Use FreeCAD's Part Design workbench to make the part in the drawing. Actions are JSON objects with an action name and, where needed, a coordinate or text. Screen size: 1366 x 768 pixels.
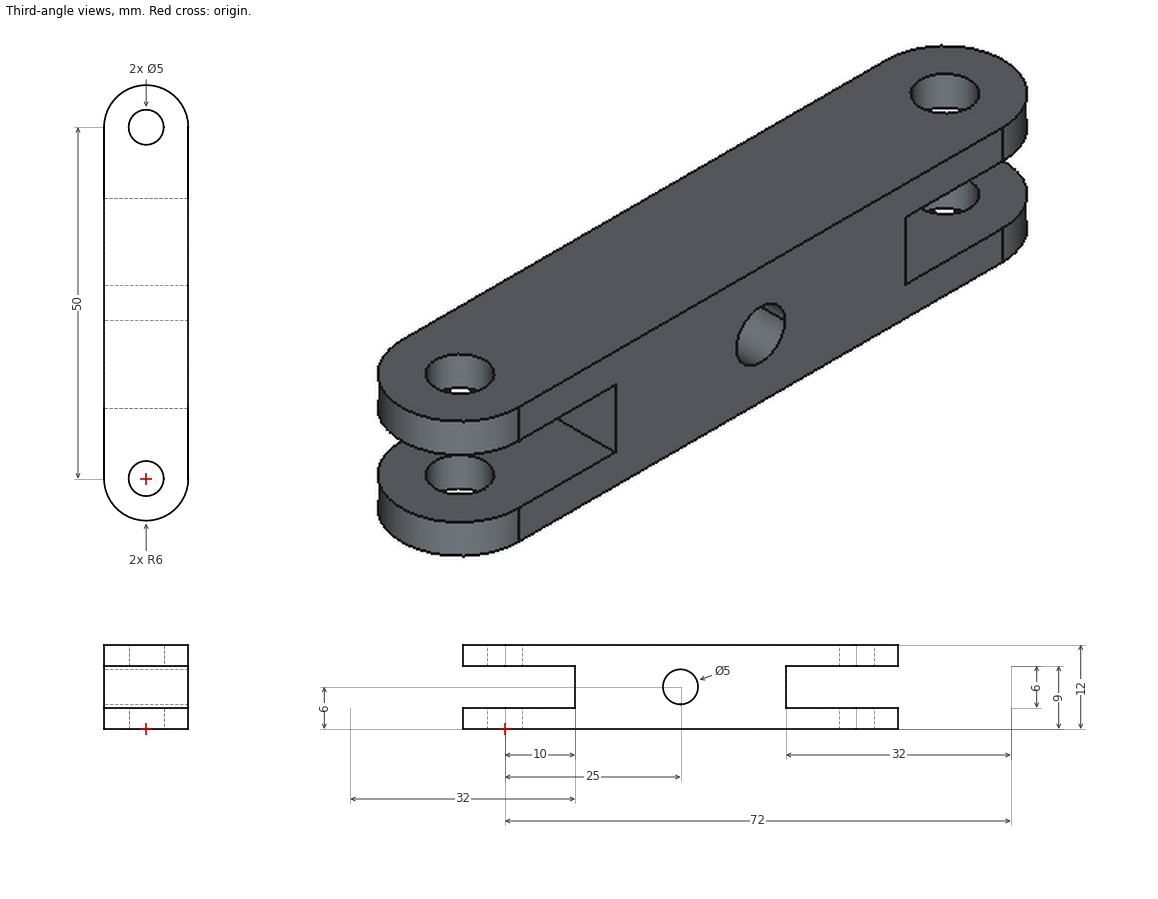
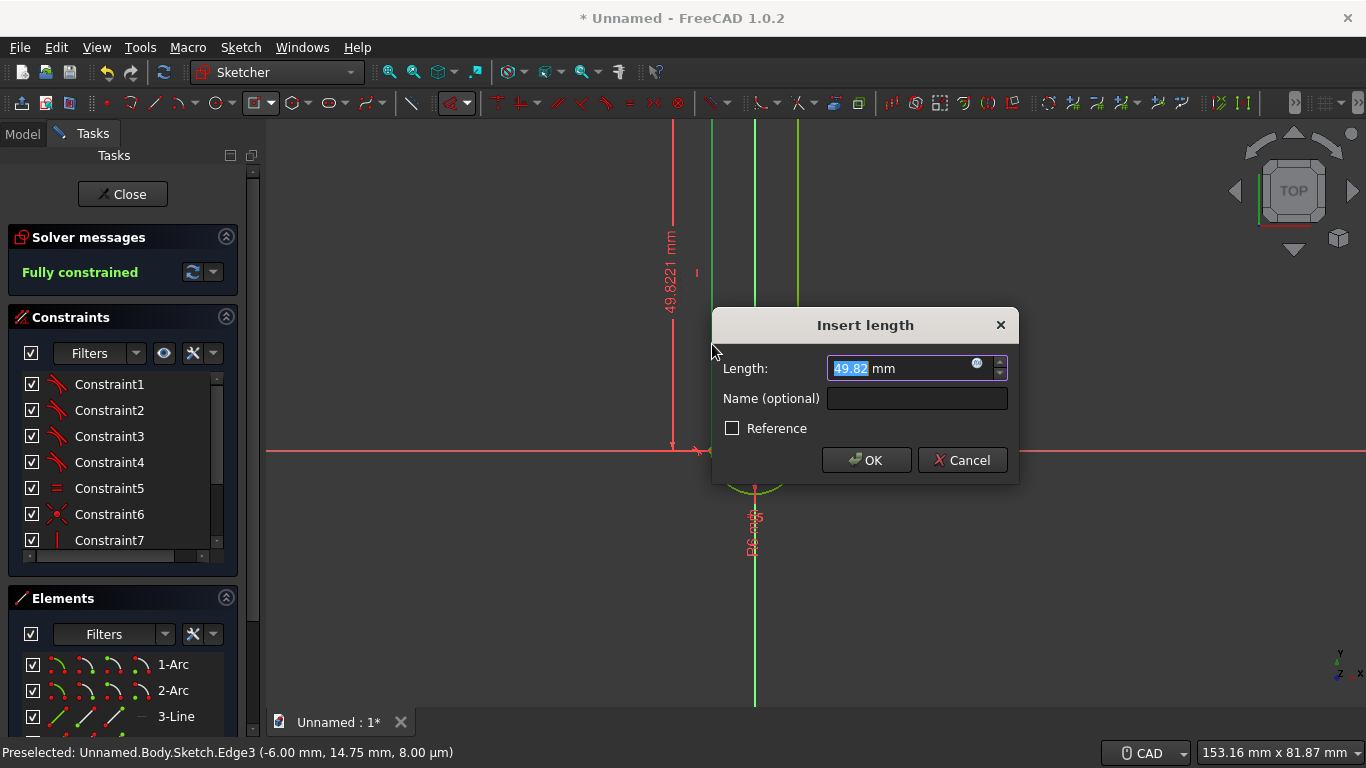
{"action": "type", "text": "50"}
{"action": "key", "text": "Return"}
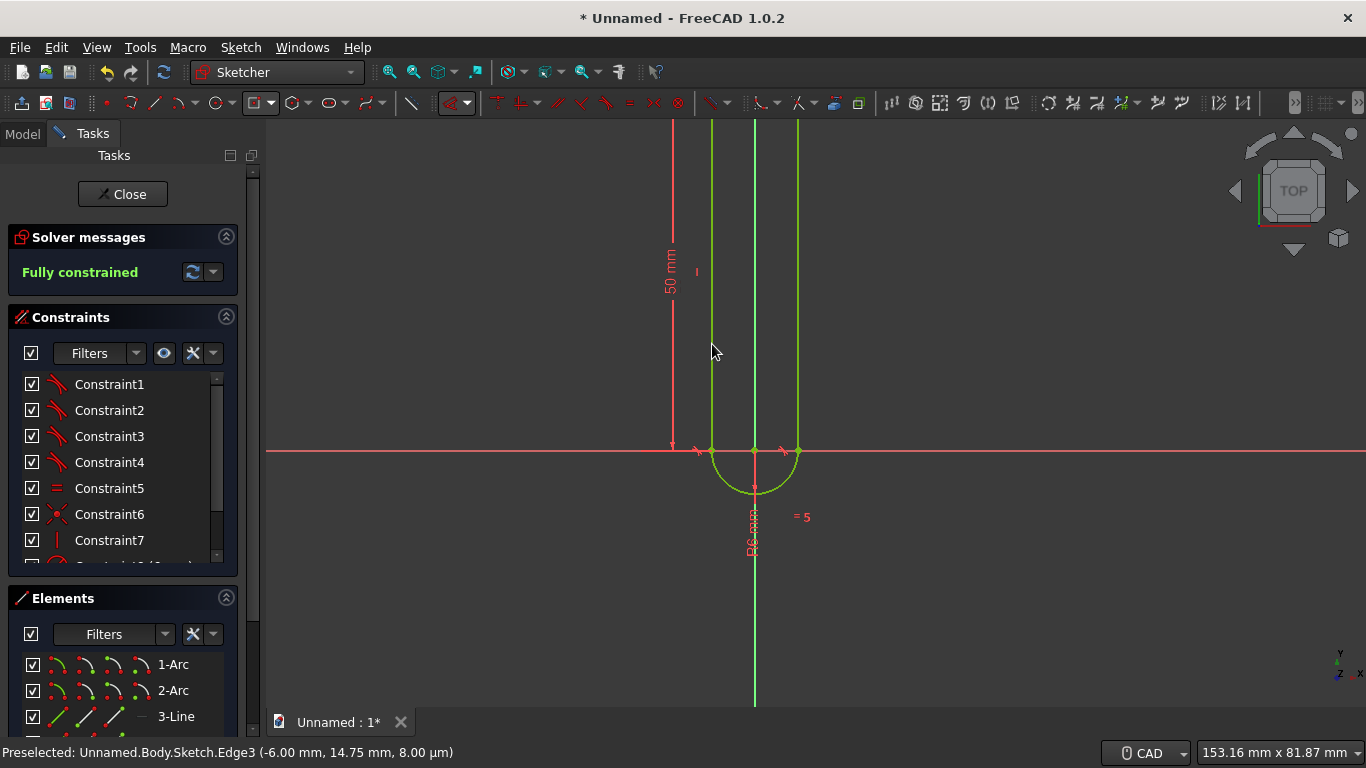
{"action": "left_click", "coordinate": [123, 194]}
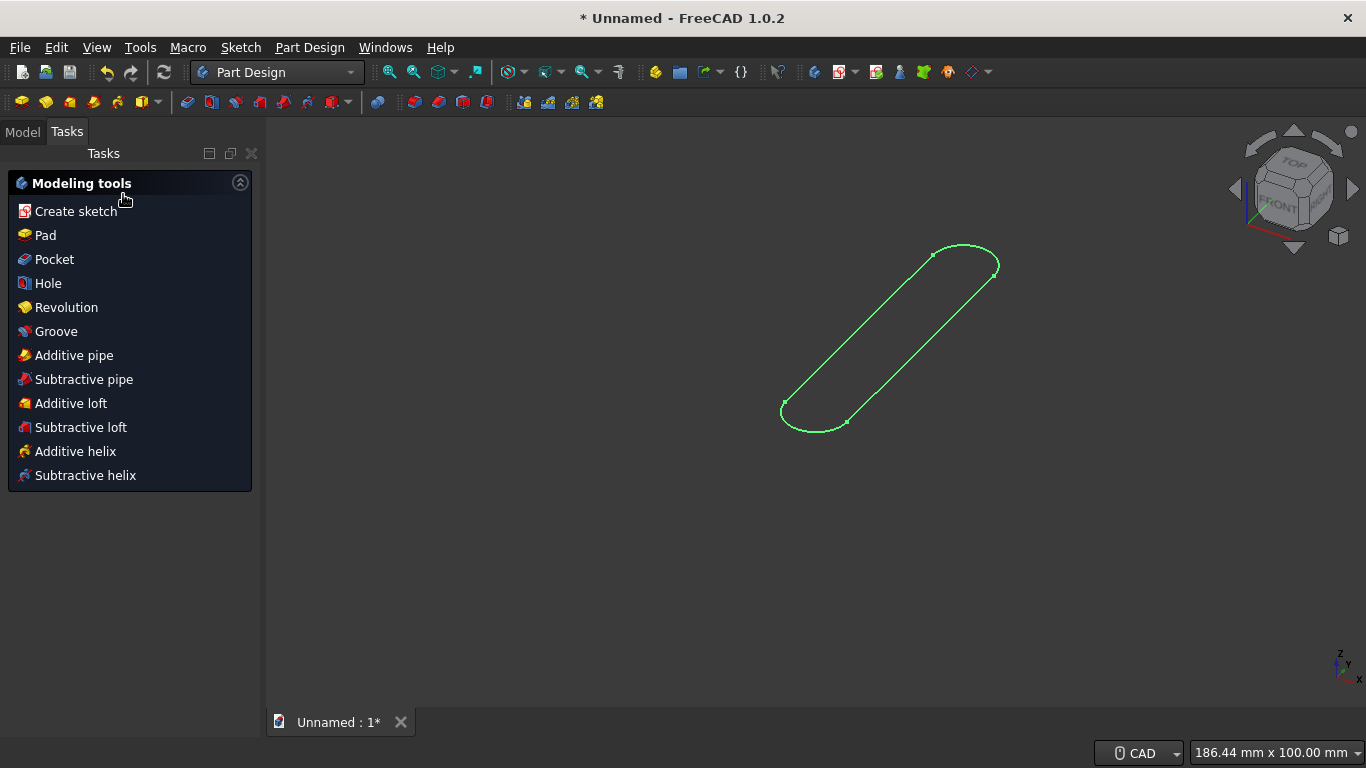
{"action": "left_click", "coordinate": [22, 102]}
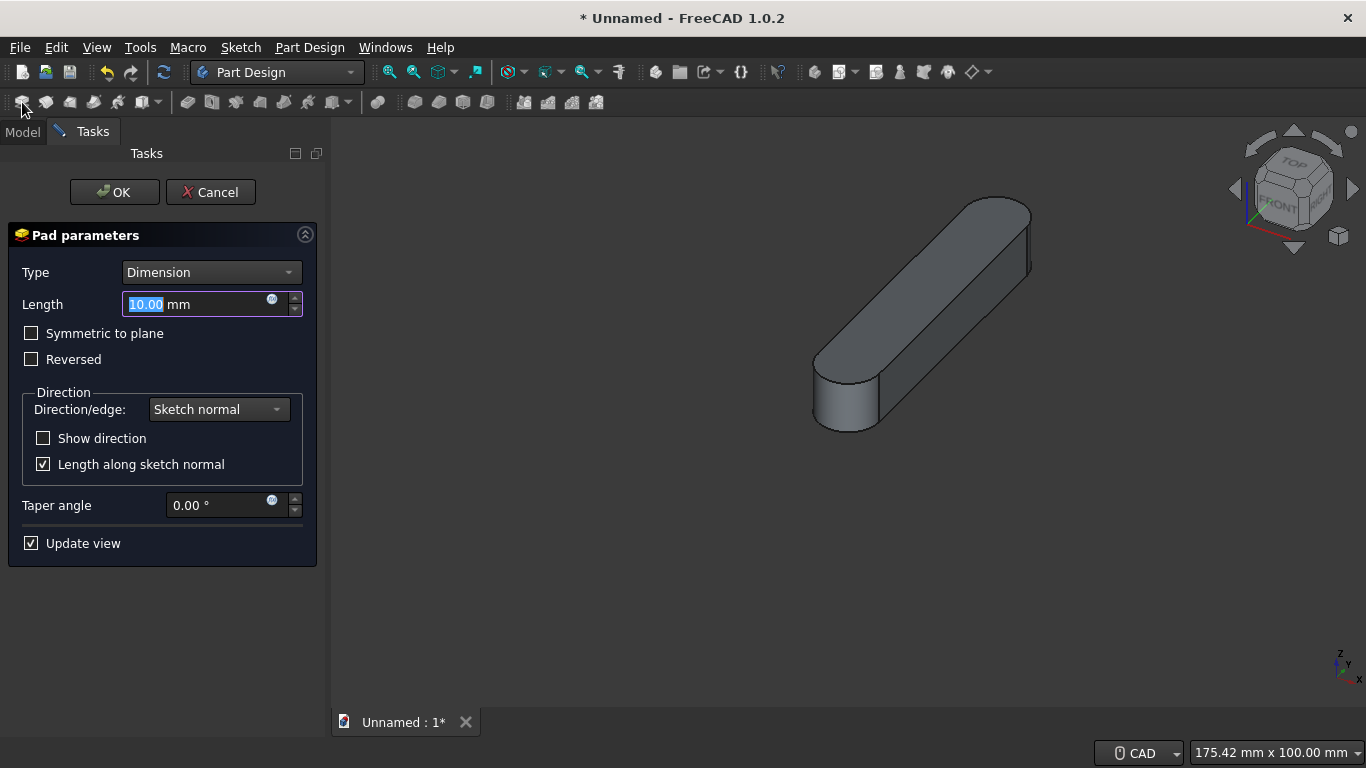
{"action": "type", "text": "12"}
{"action": "key", "text": "Tab"}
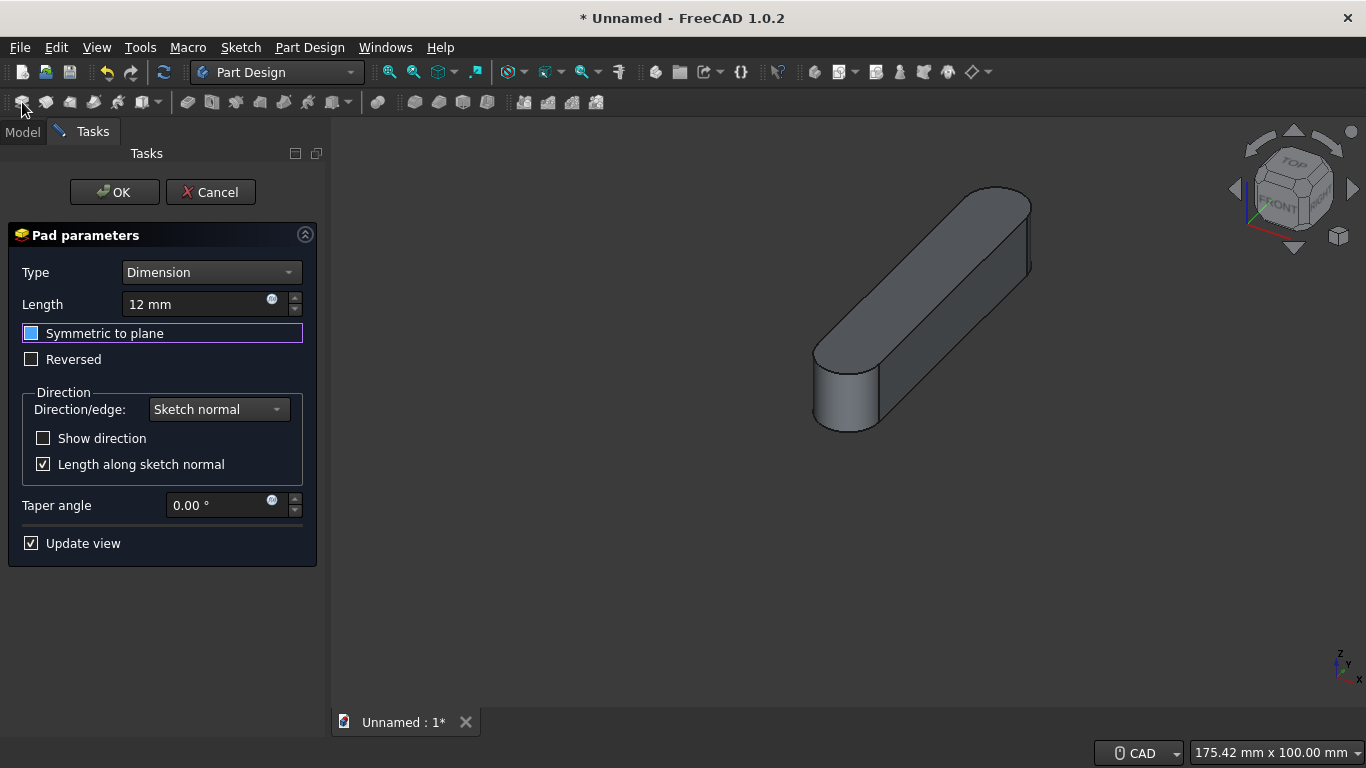
{"action": "left_click", "coordinate": [115, 192]}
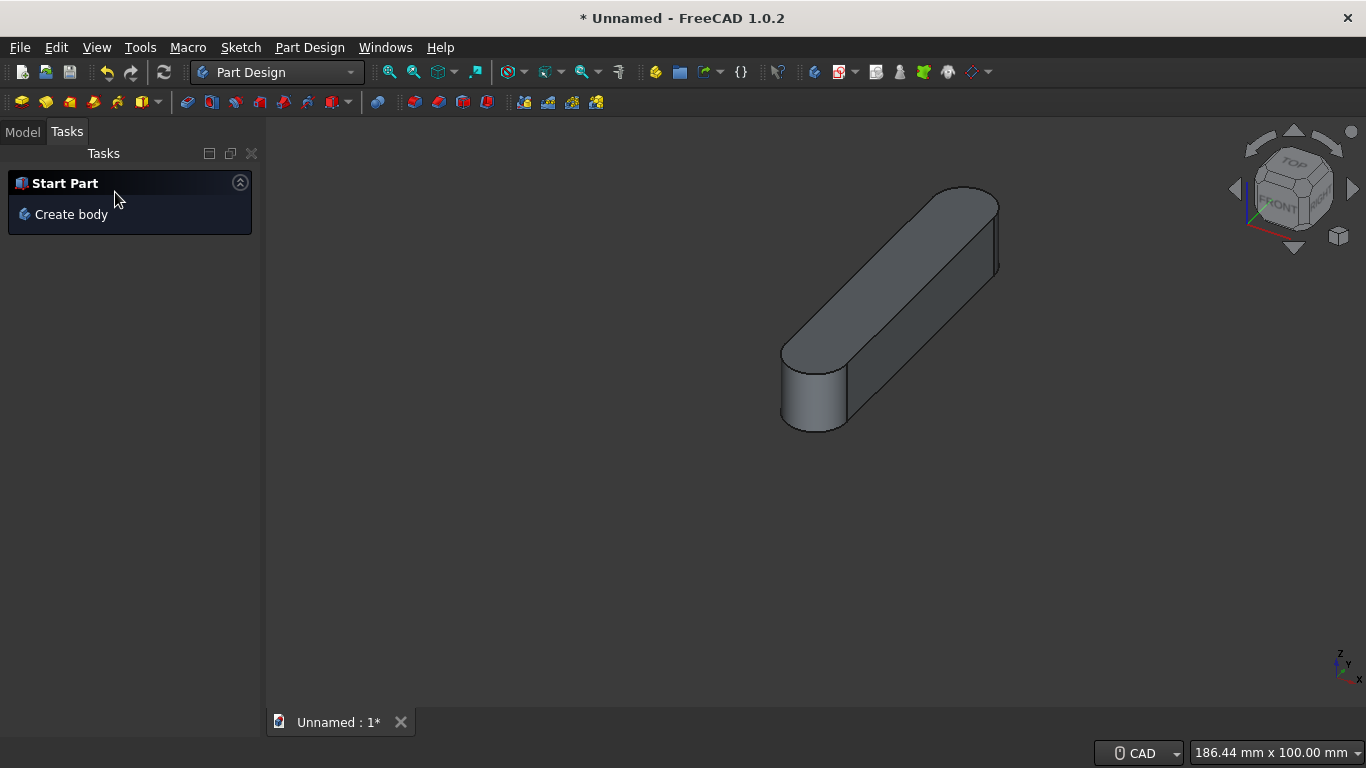
{"action": "left_click", "coordinate": [390, 72]}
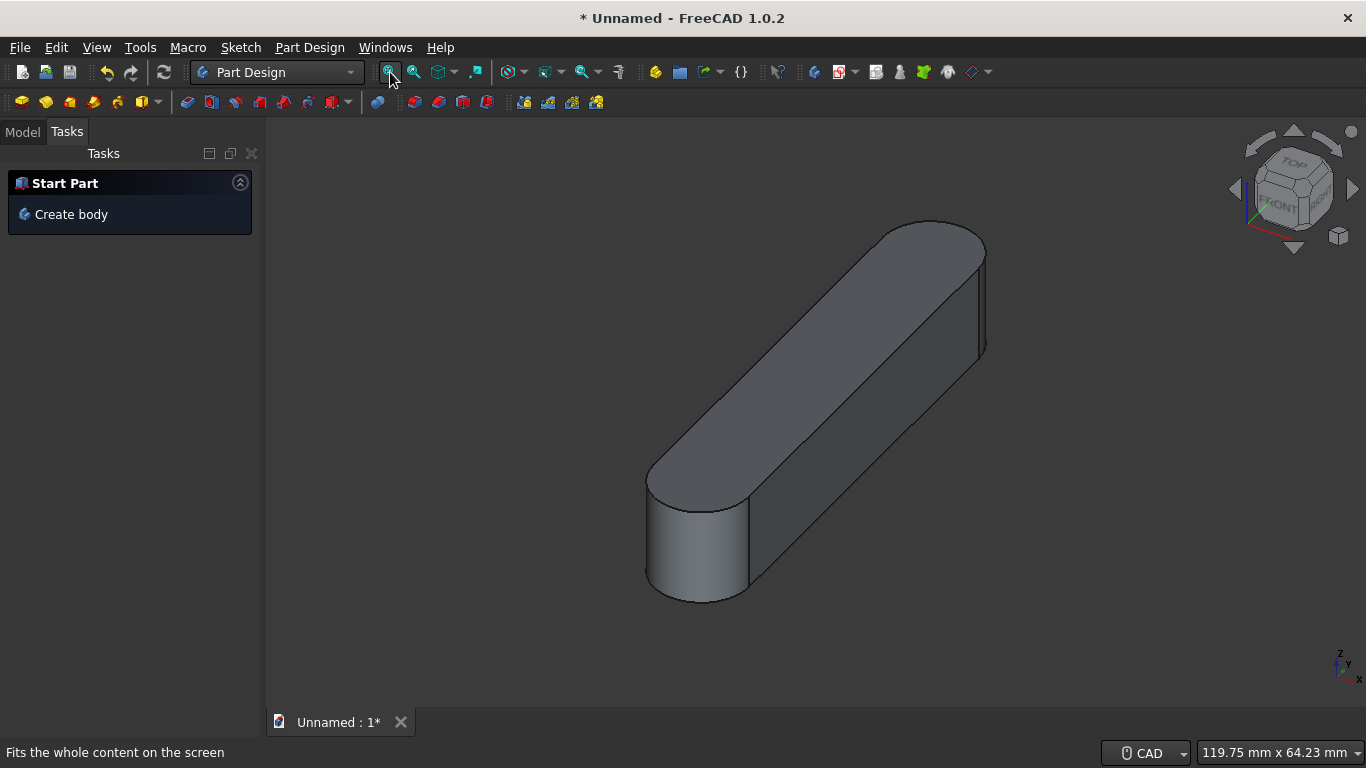
{"action": "key", "text": "6"}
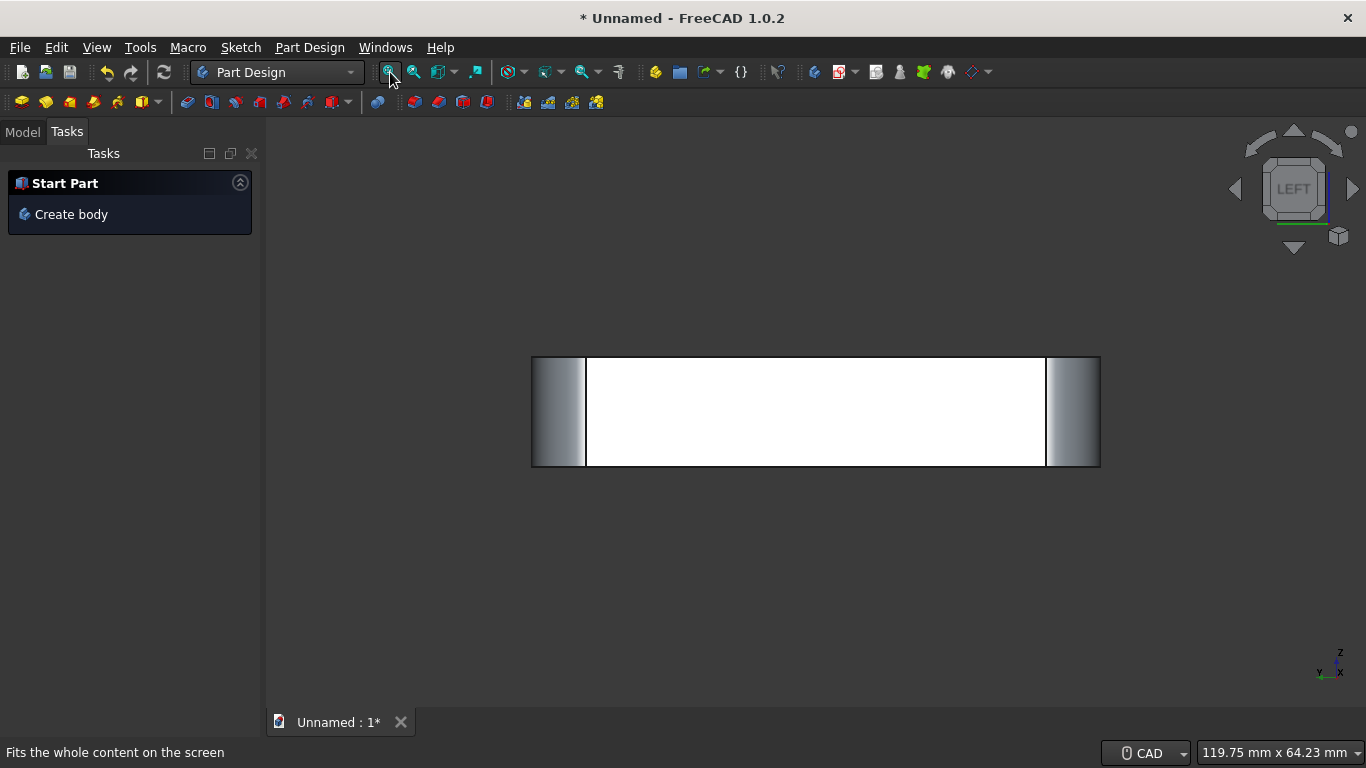
{"action": "left_click", "coordinate": [685, 411]}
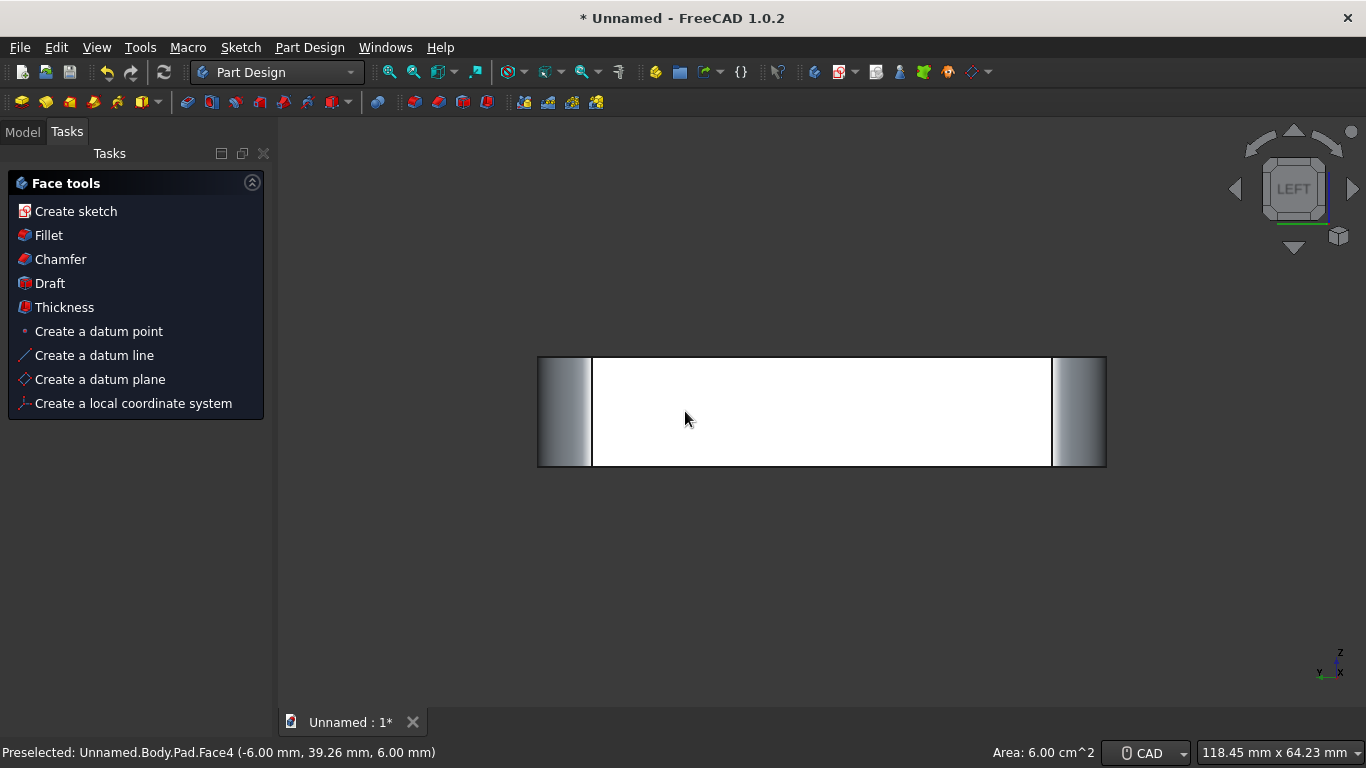
{"action": "left_click", "coordinate": [840, 72]}